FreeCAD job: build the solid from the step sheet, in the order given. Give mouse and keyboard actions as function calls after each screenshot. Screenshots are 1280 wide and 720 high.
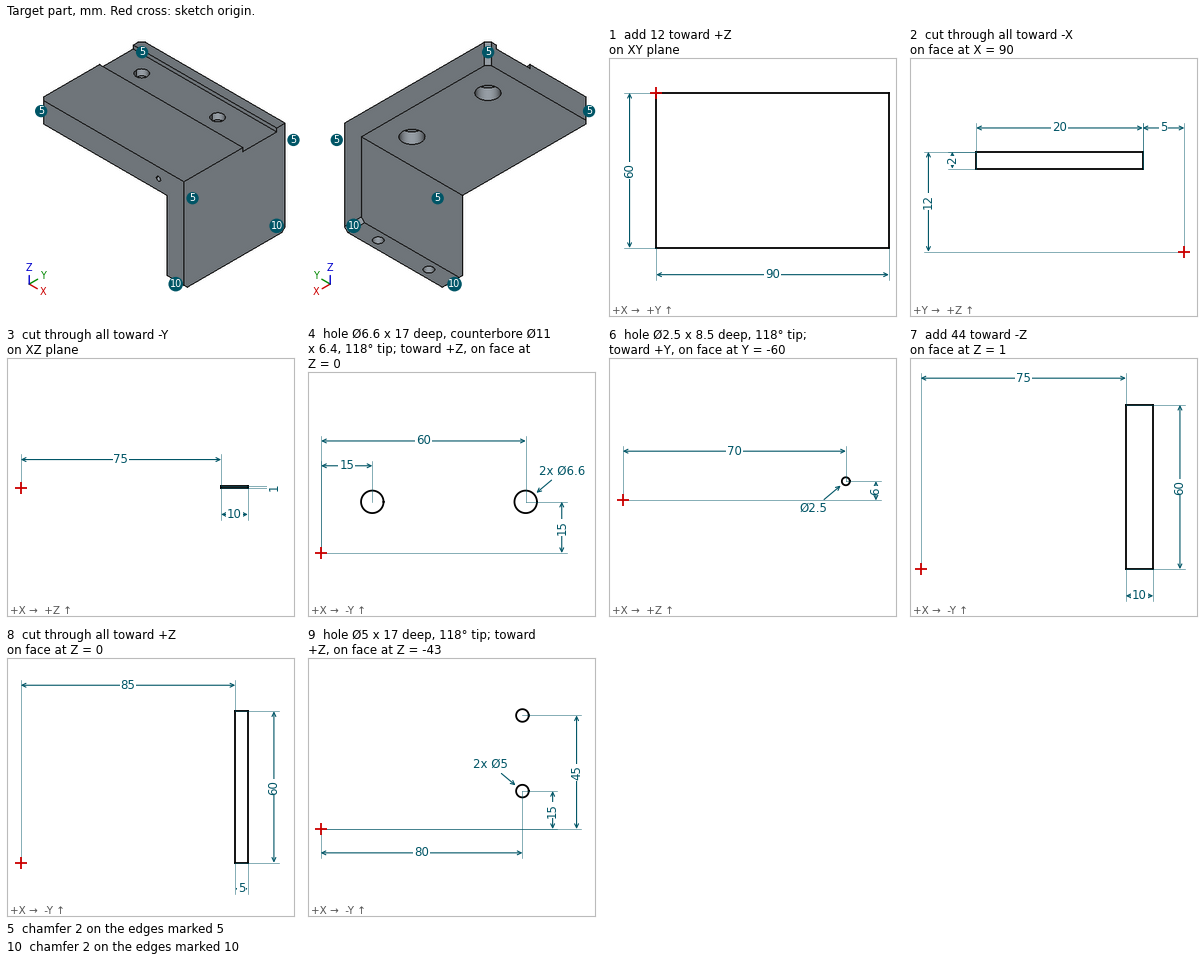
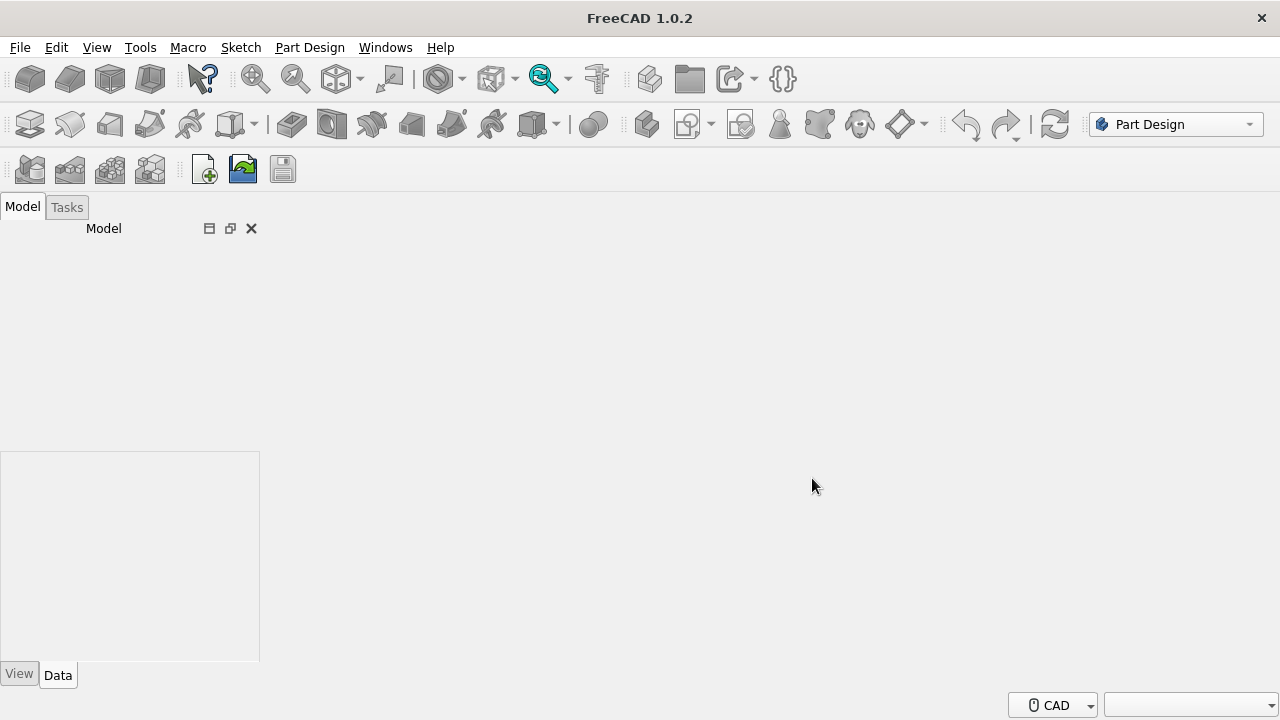
click(204, 170)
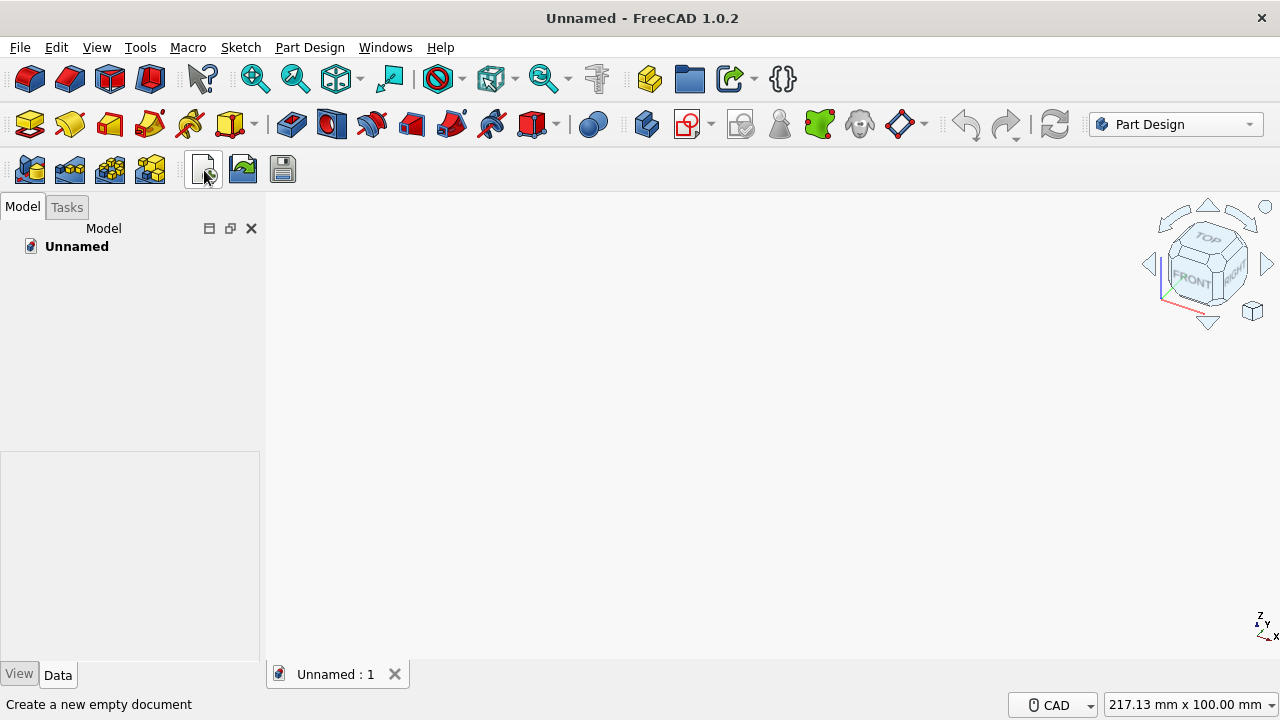
click(688, 124)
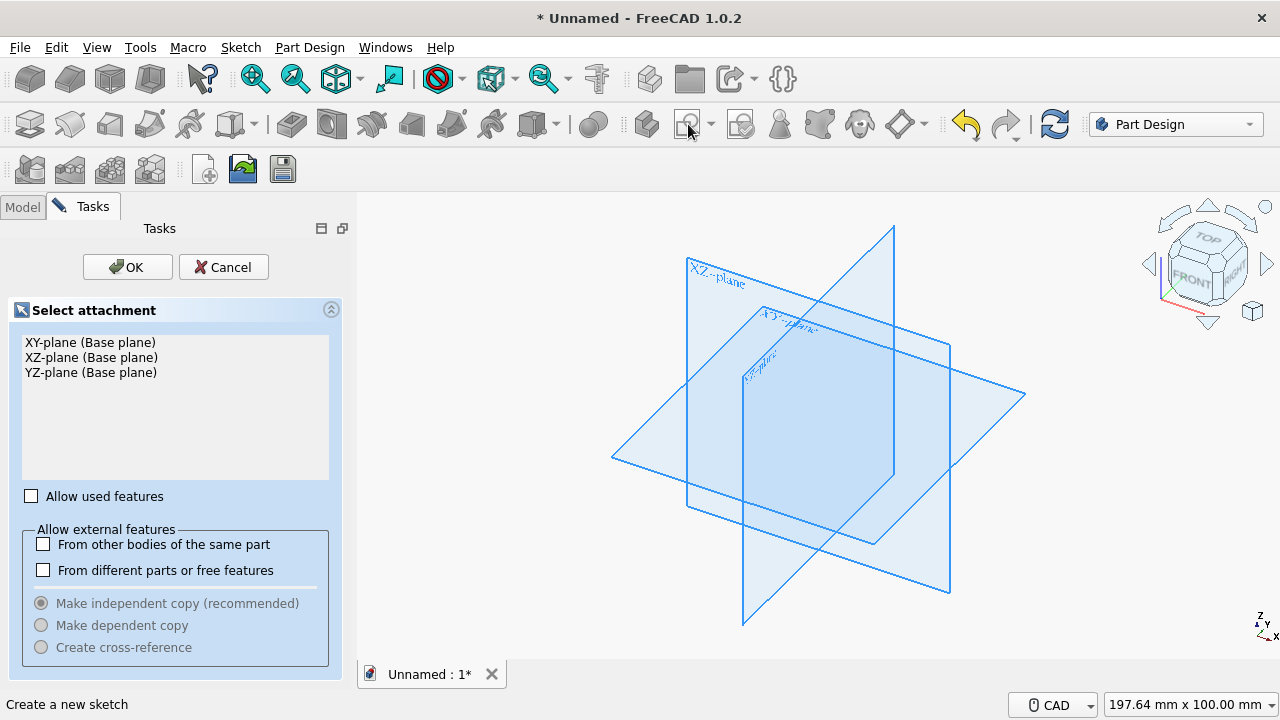
click(82, 342)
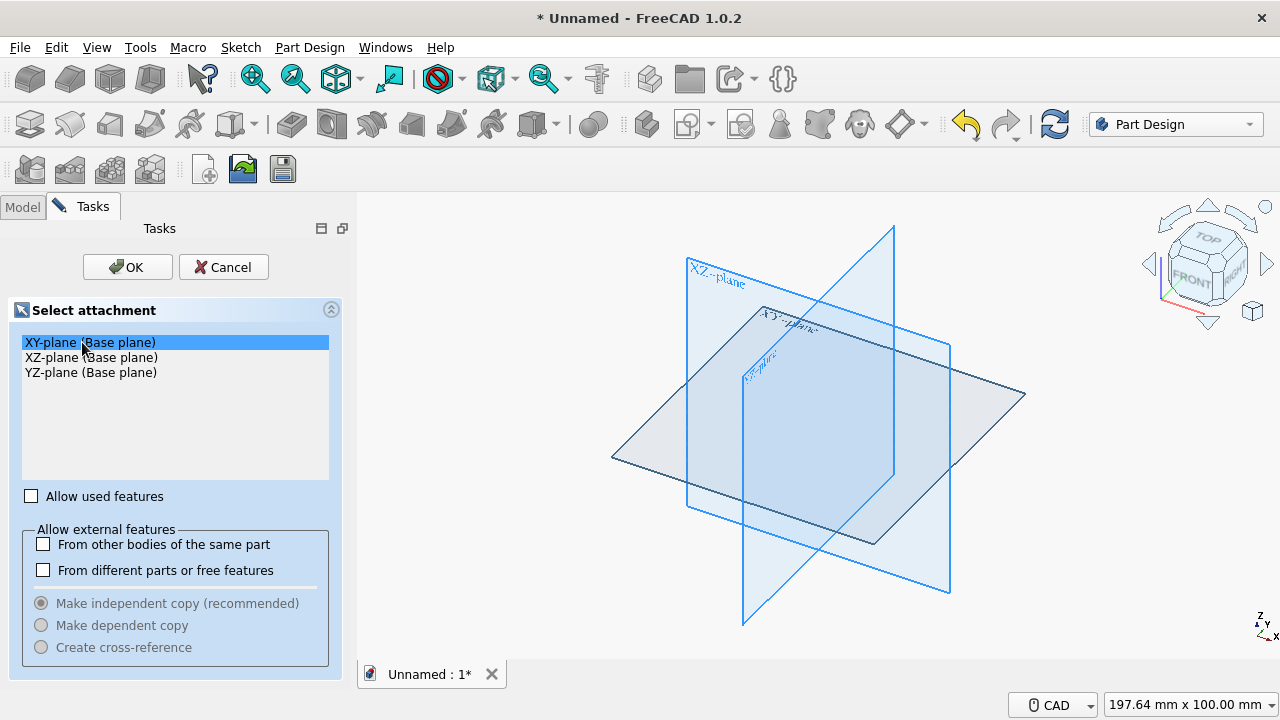
click(128, 267)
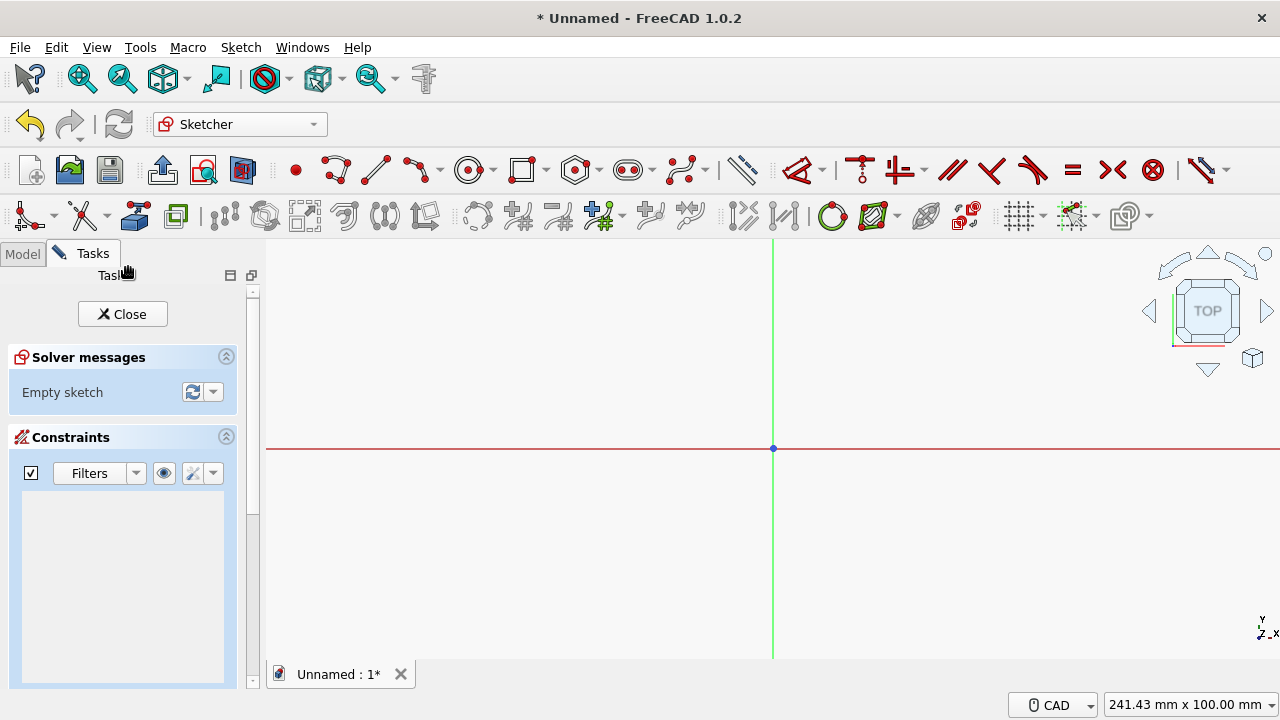
scroll(294, 267, down, 2)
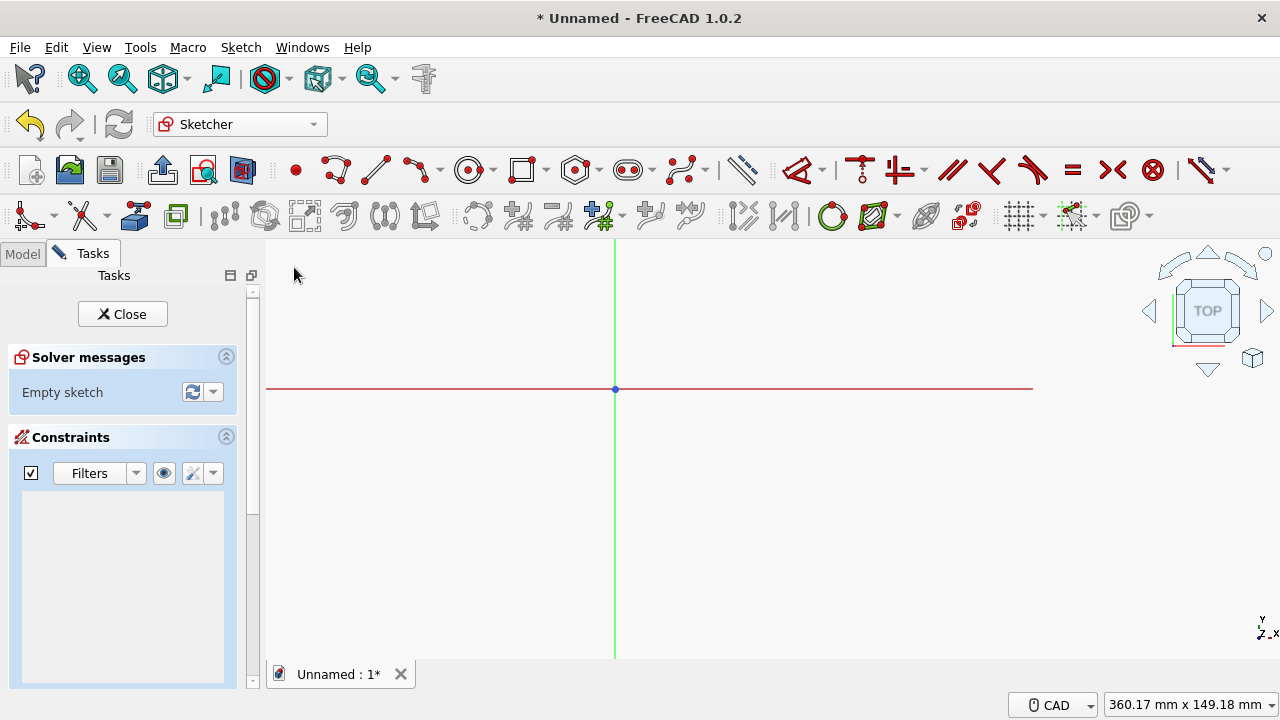
scroll(818, 523, up, 2)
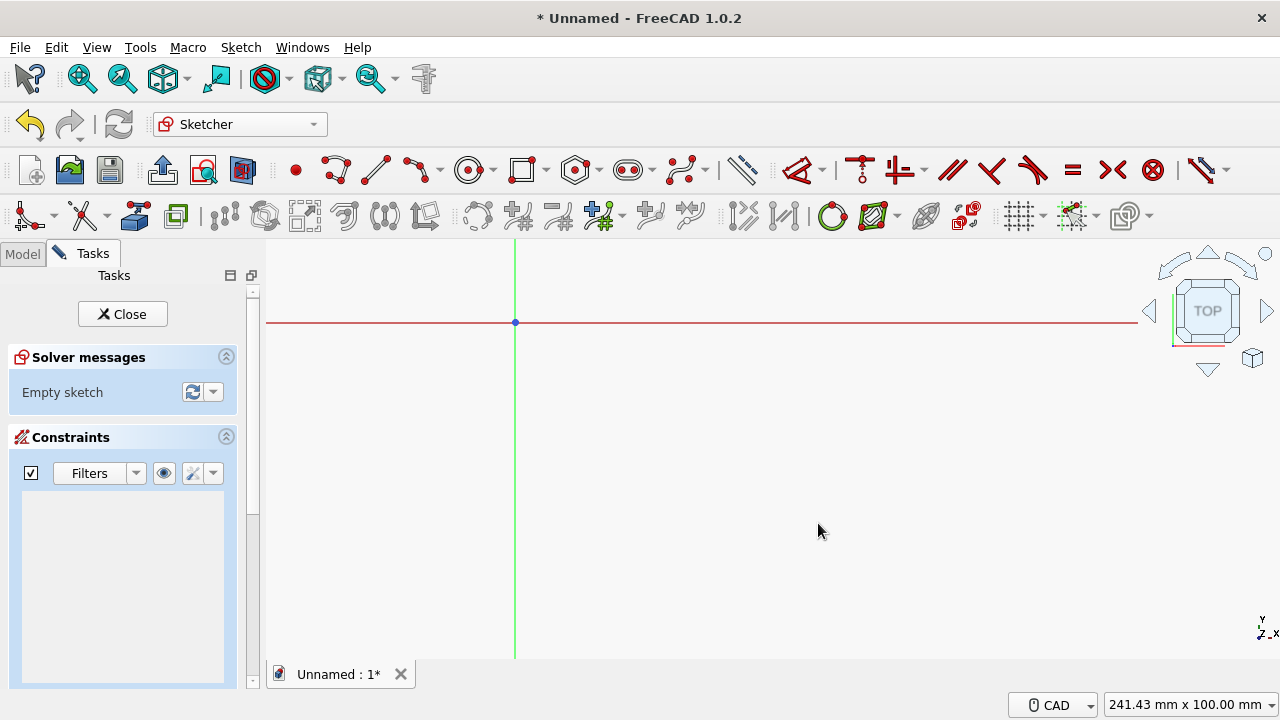
click(522, 170)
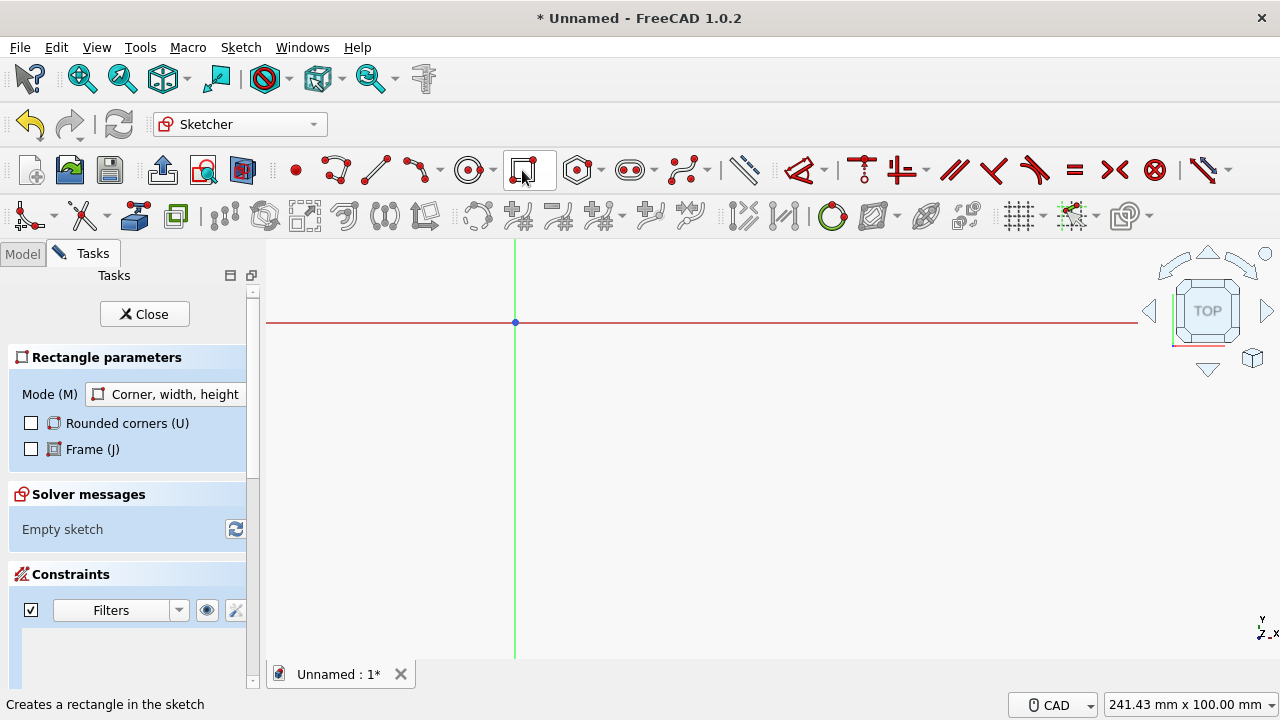
click(515, 323)
click(893, 575)
key(Escape)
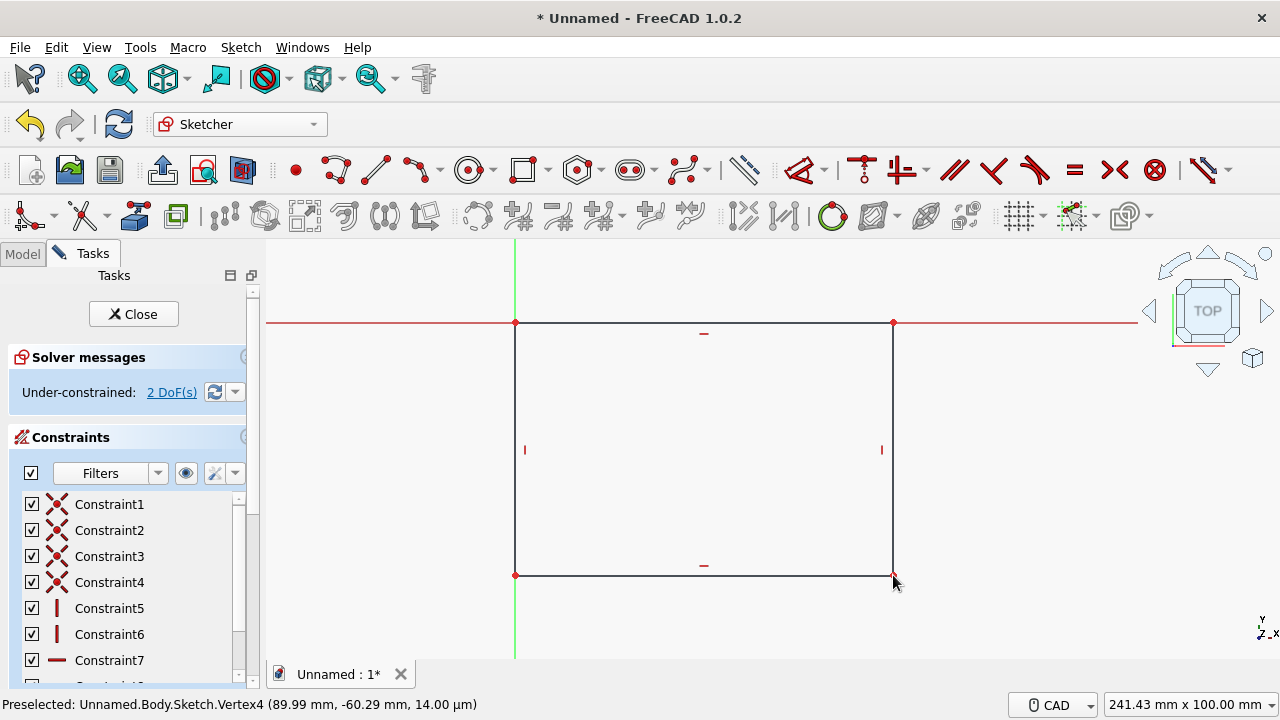
click(800, 170)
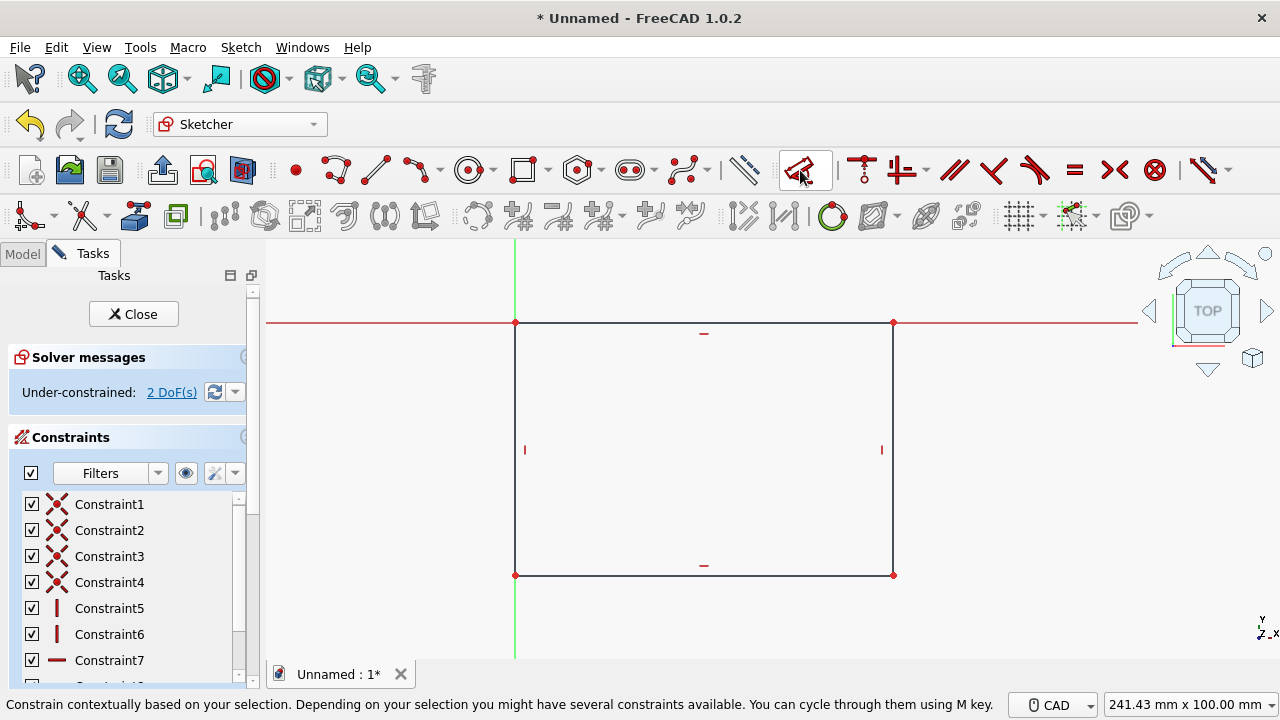
click(515, 399)
click(481, 449)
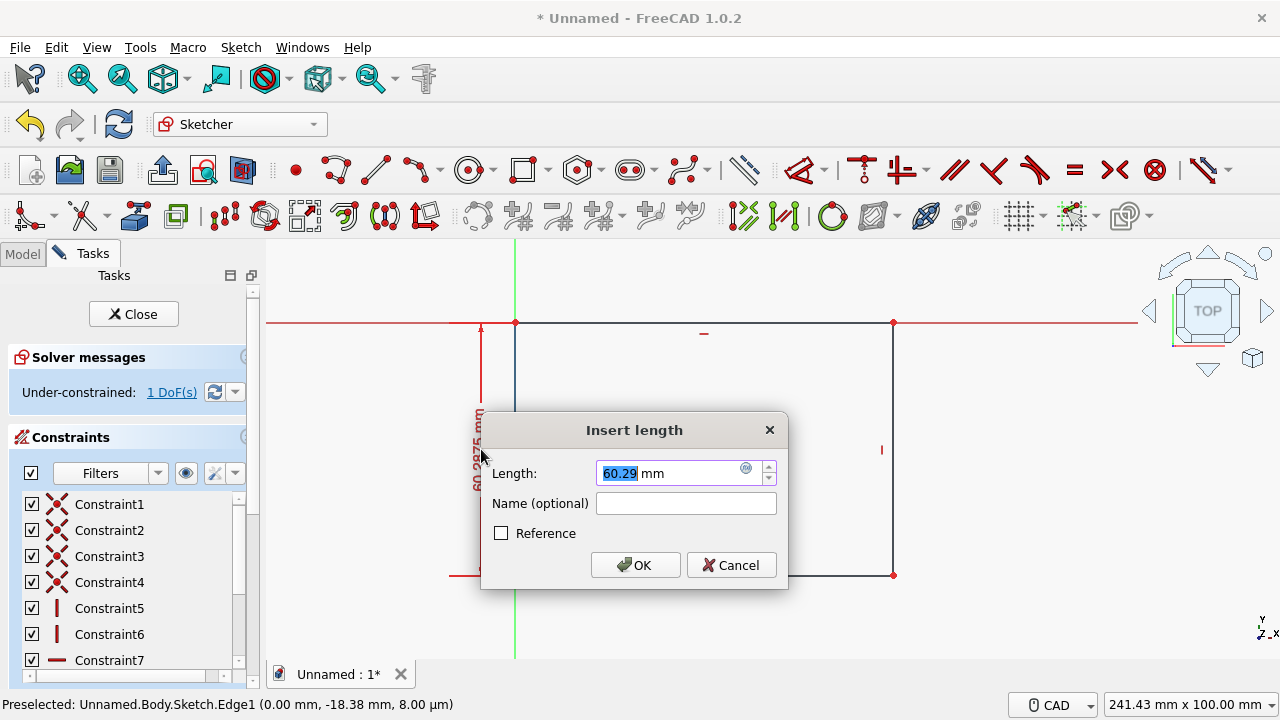
text(60)
key(Return)